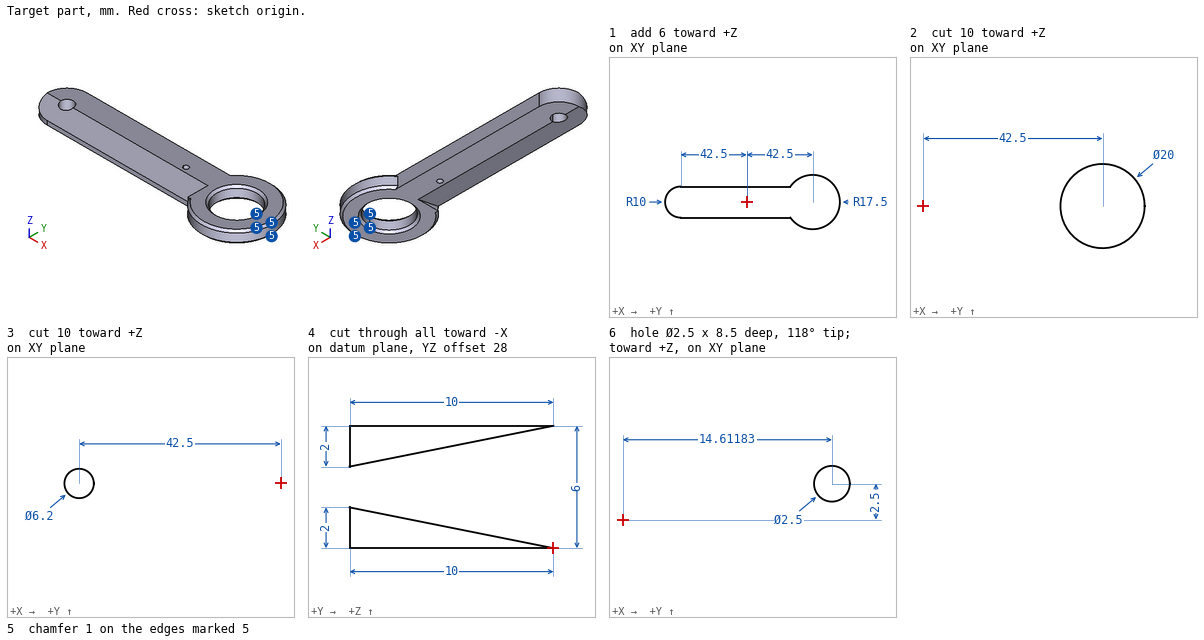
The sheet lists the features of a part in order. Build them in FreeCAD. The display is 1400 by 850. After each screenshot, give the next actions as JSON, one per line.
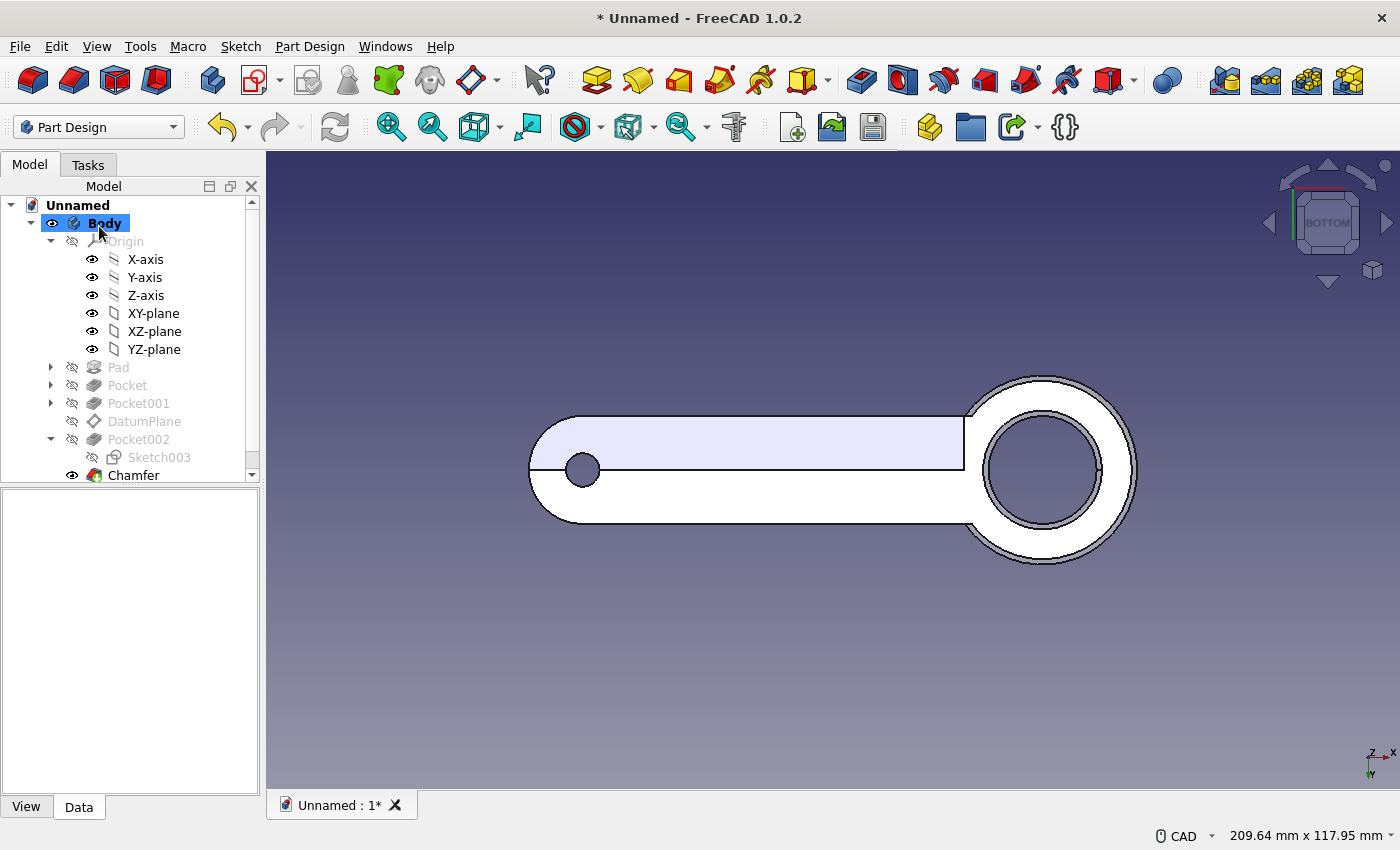
{"action": "left_click", "coordinate": [254, 80]}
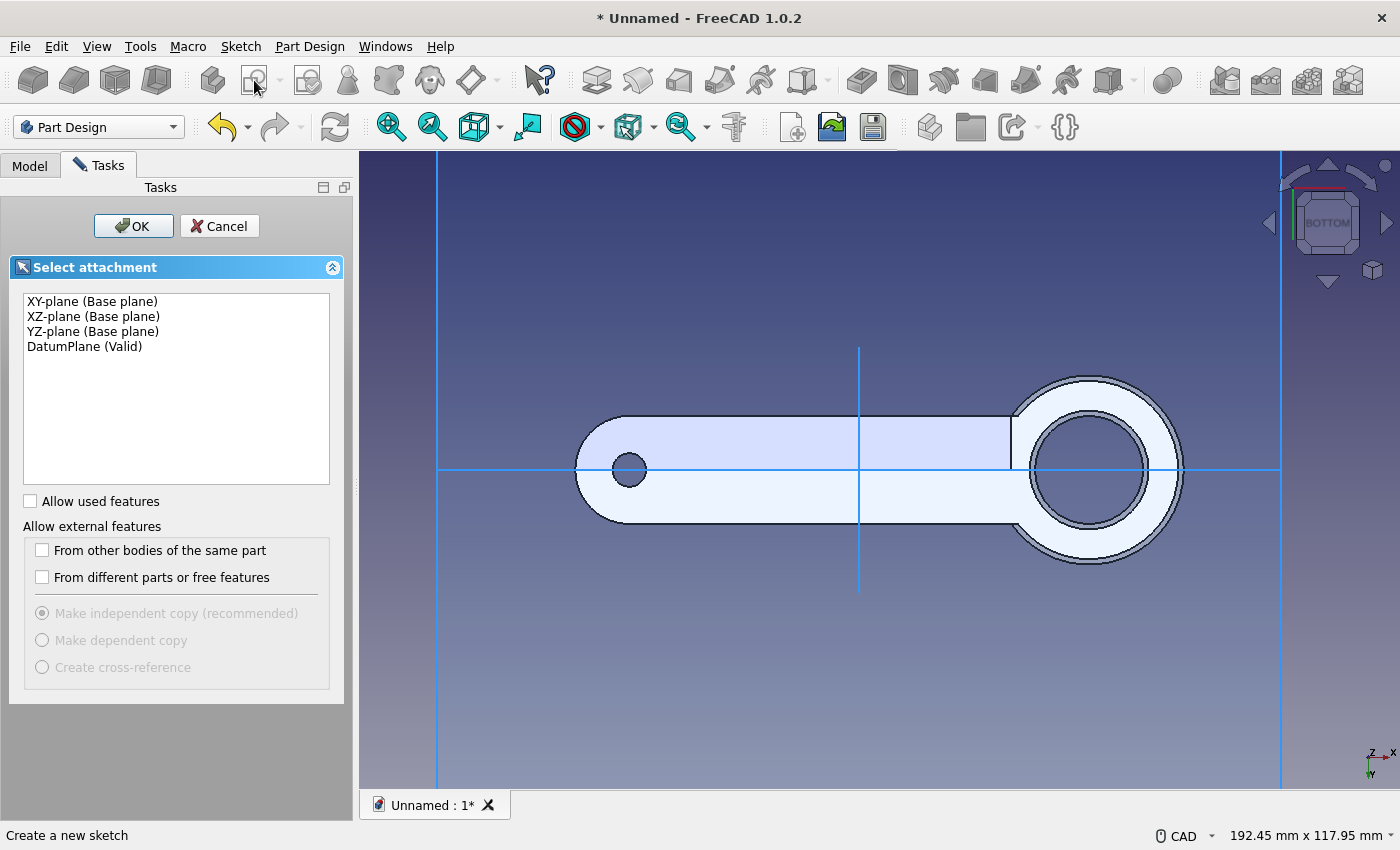
{"action": "left_click", "coordinate": [84, 302]}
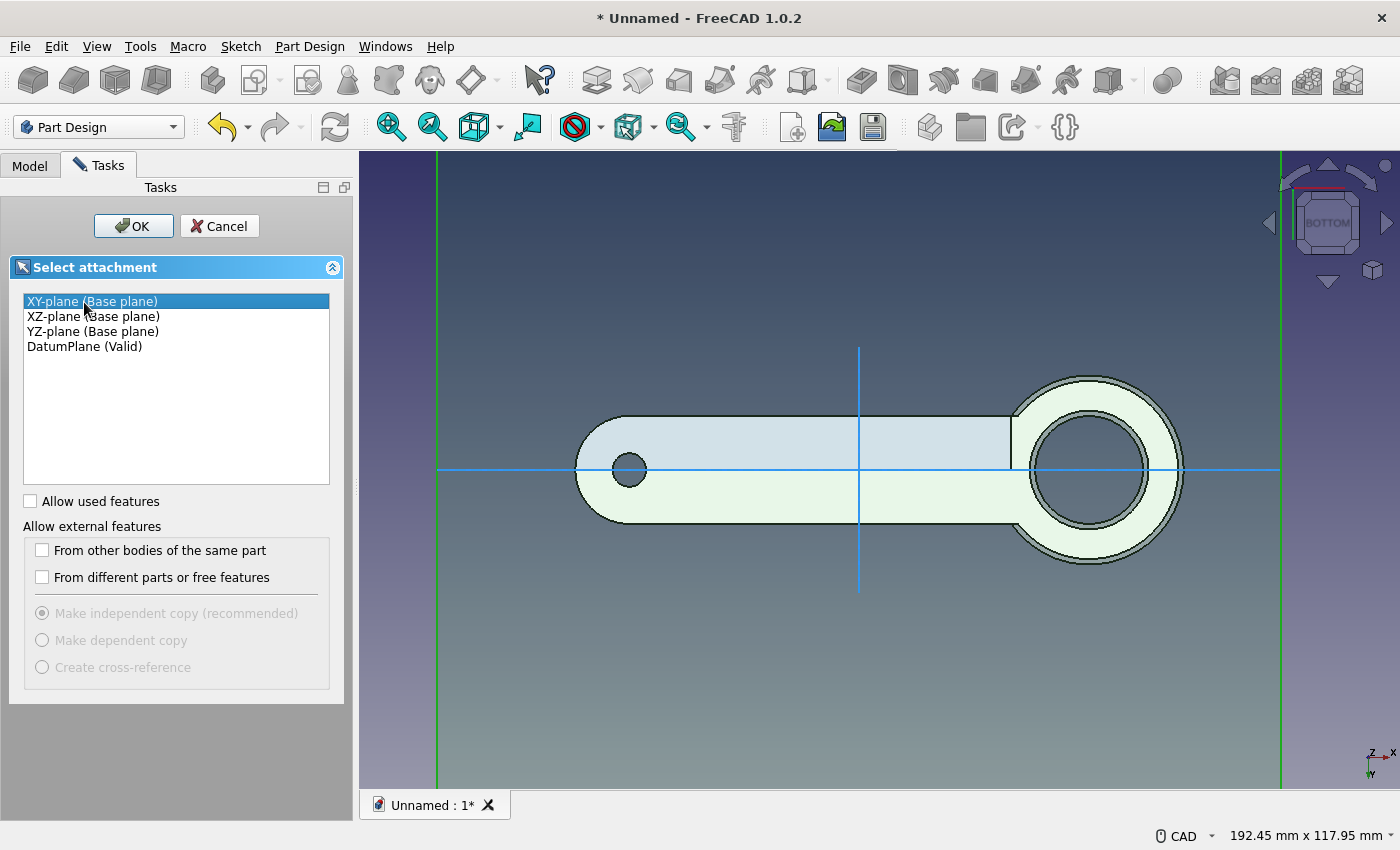
{"action": "left_click", "coordinate": [134, 226]}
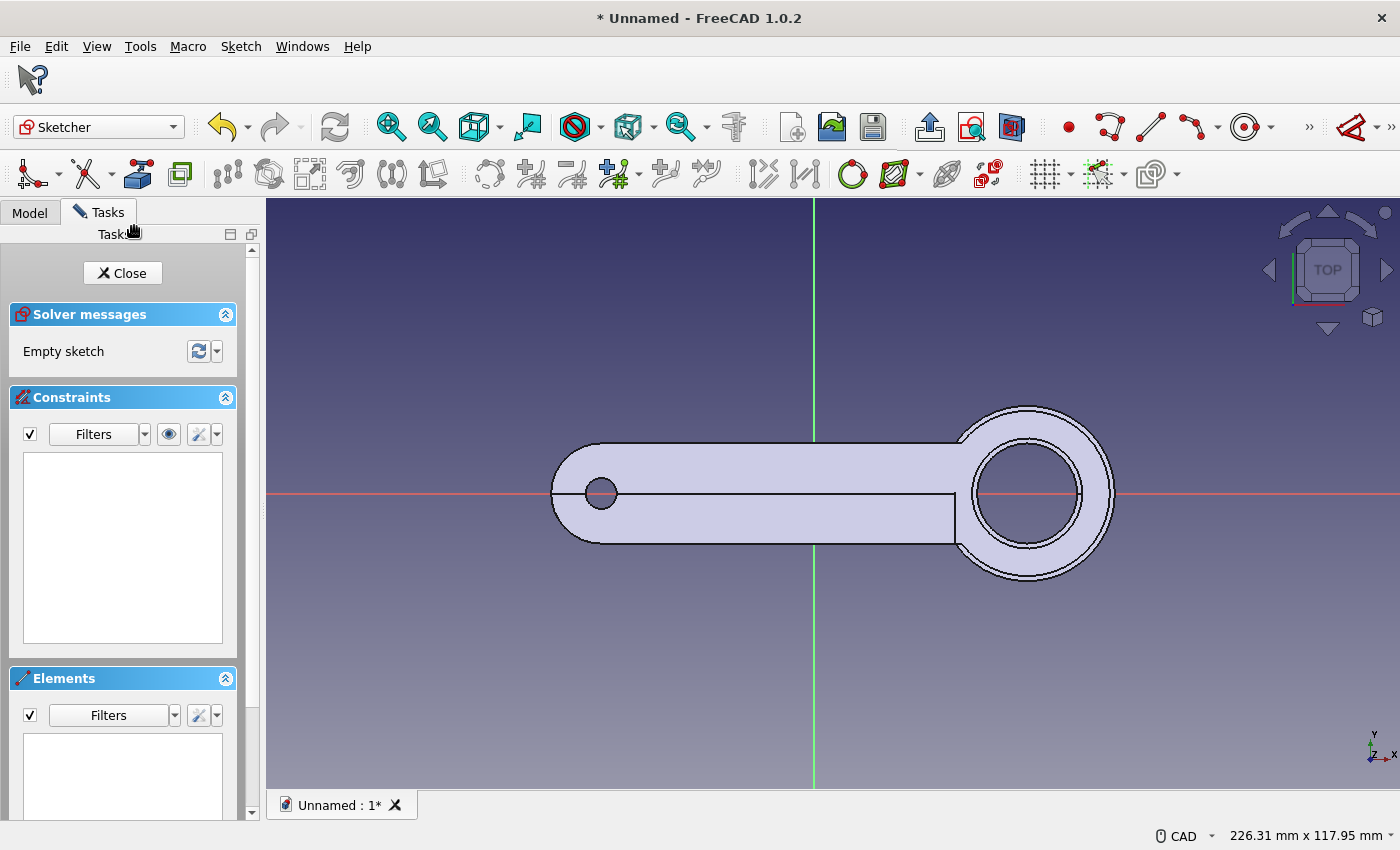
{"action": "key", "text": "q s"}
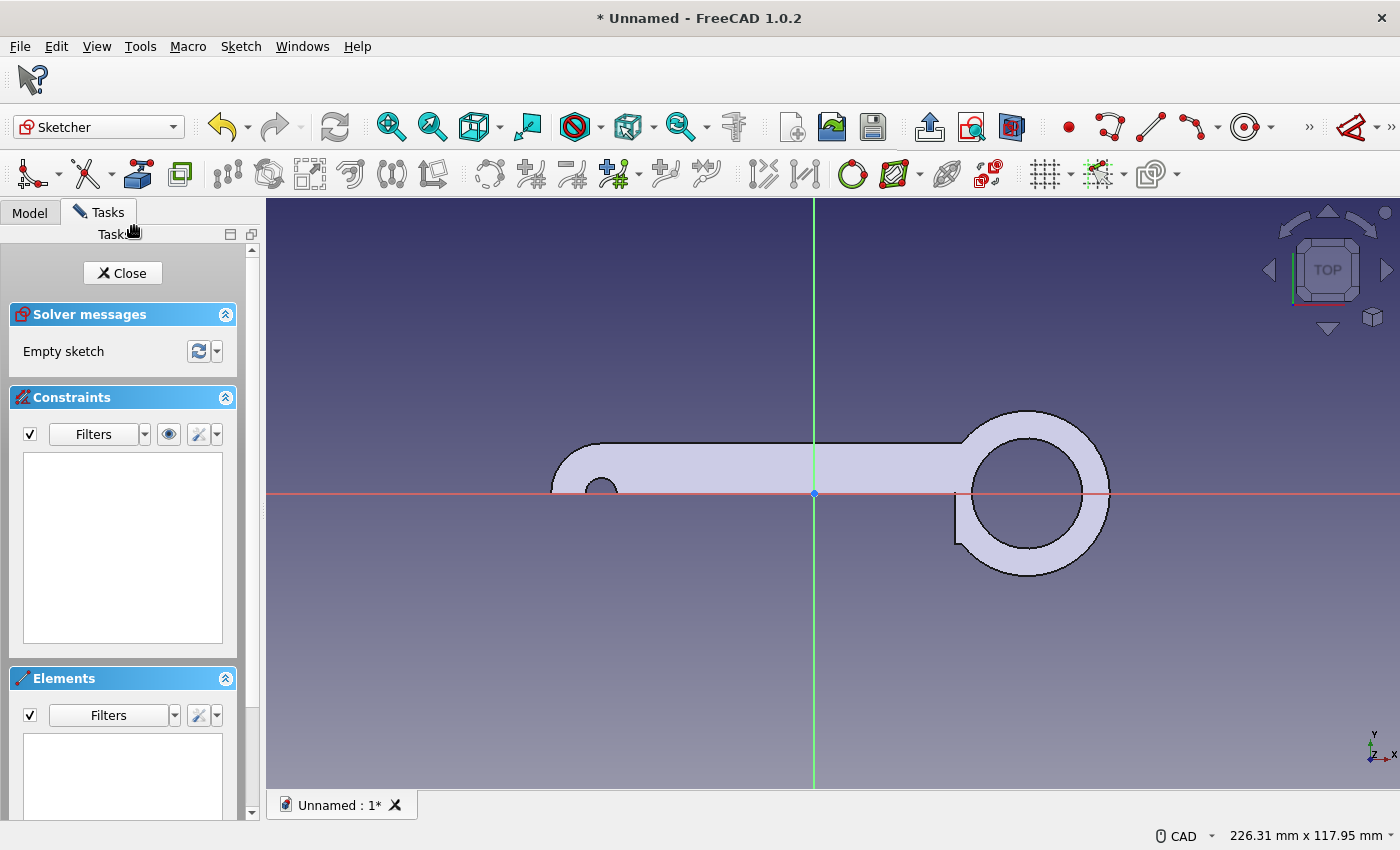
{"action": "scroll", "coordinate": [894, 480], "scroll_direction": "up", "scroll_amount": 15}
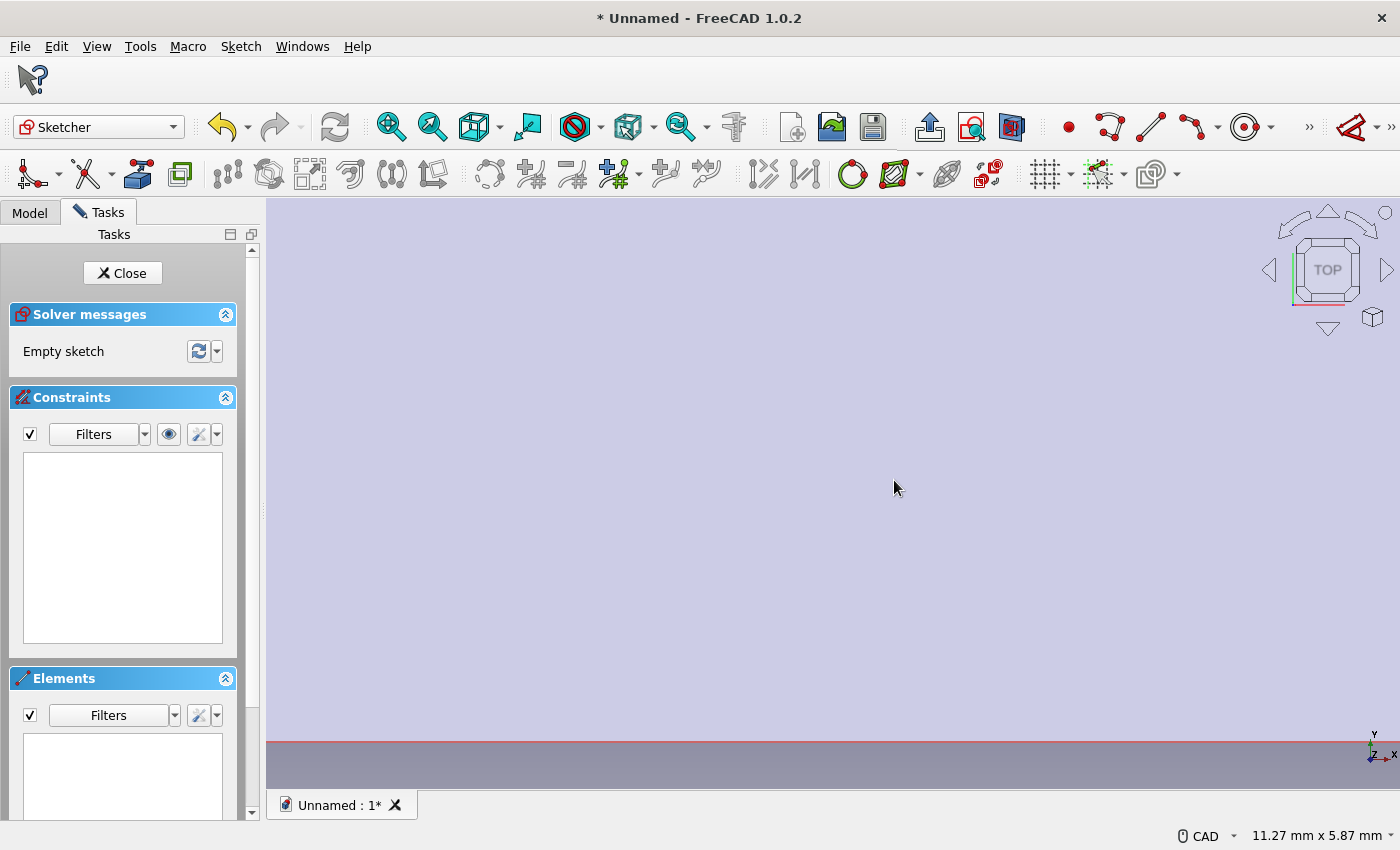
{"action": "scroll", "coordinate": [725, 484], "scroll_direction": "up", "scroll_amount": 2}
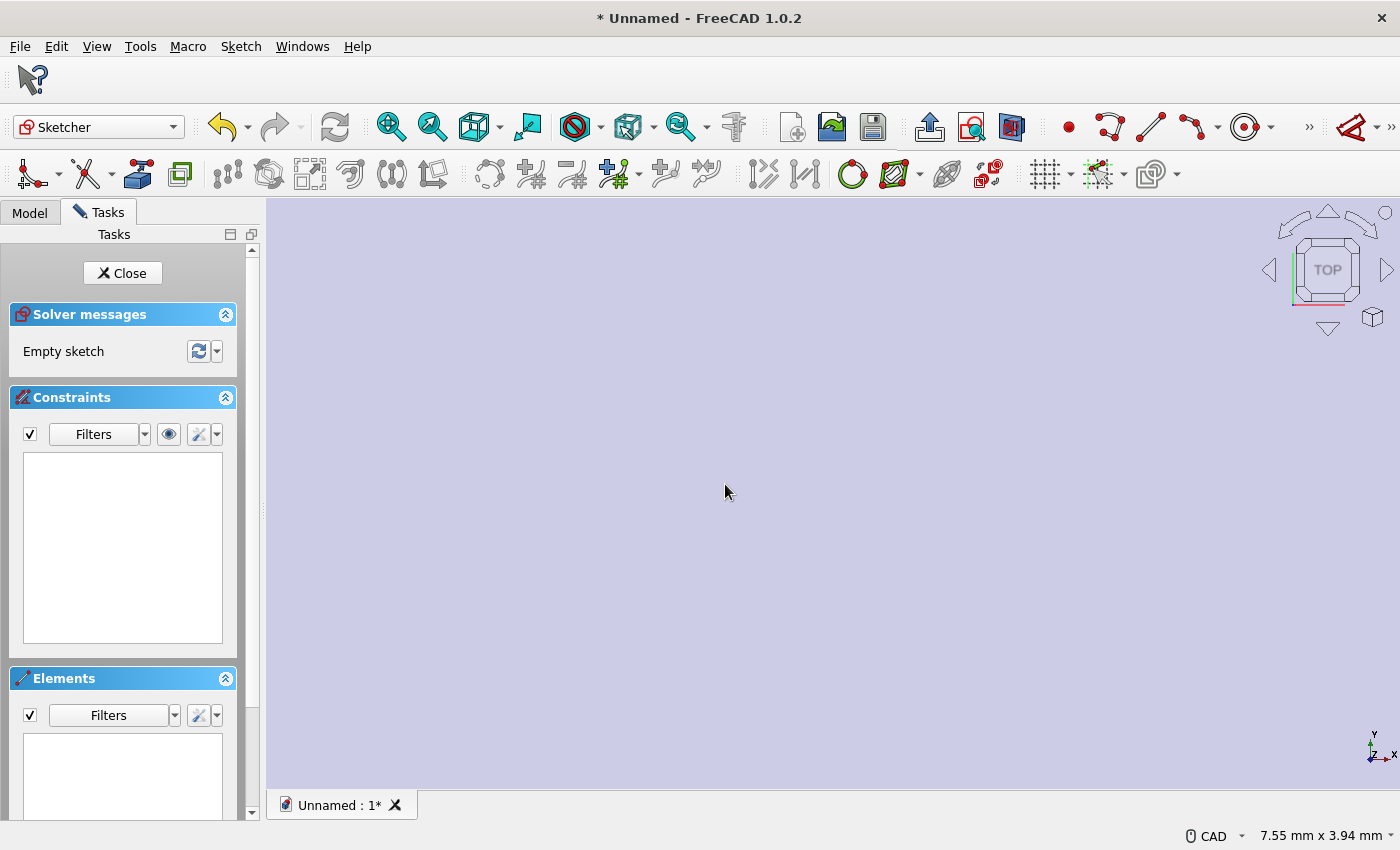
{"action": "key", "text": "g c"}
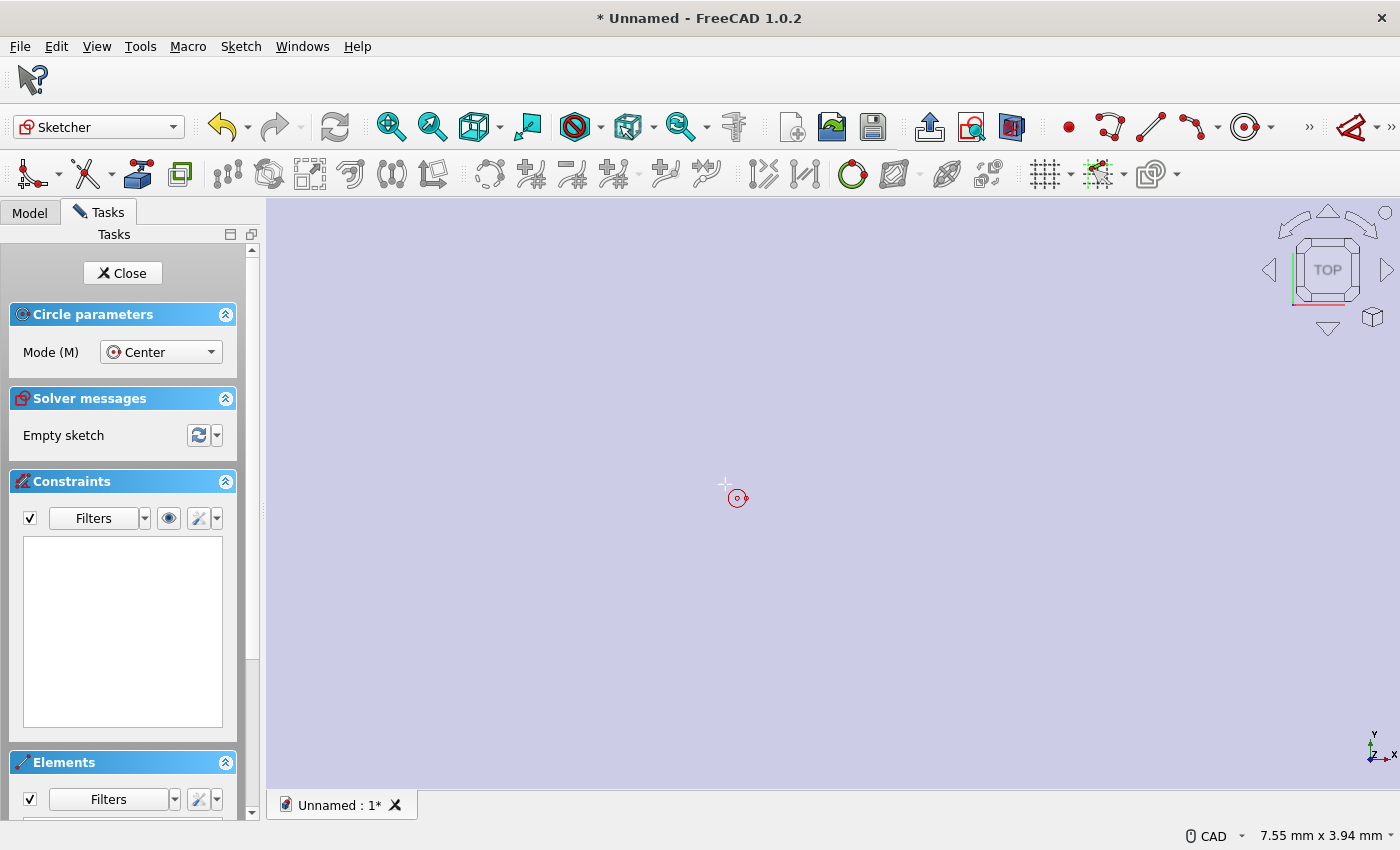
{"action": "left_click", "coordinate": [764, 493]}
{"action": "left_click", "coordinate": [897, 361]}
{"action": "key", "text": "Escape"}